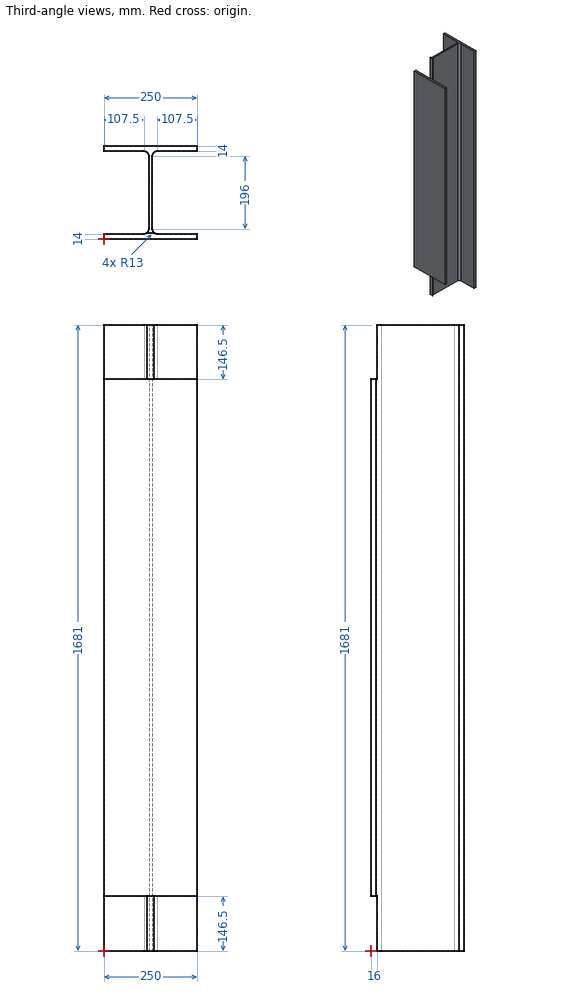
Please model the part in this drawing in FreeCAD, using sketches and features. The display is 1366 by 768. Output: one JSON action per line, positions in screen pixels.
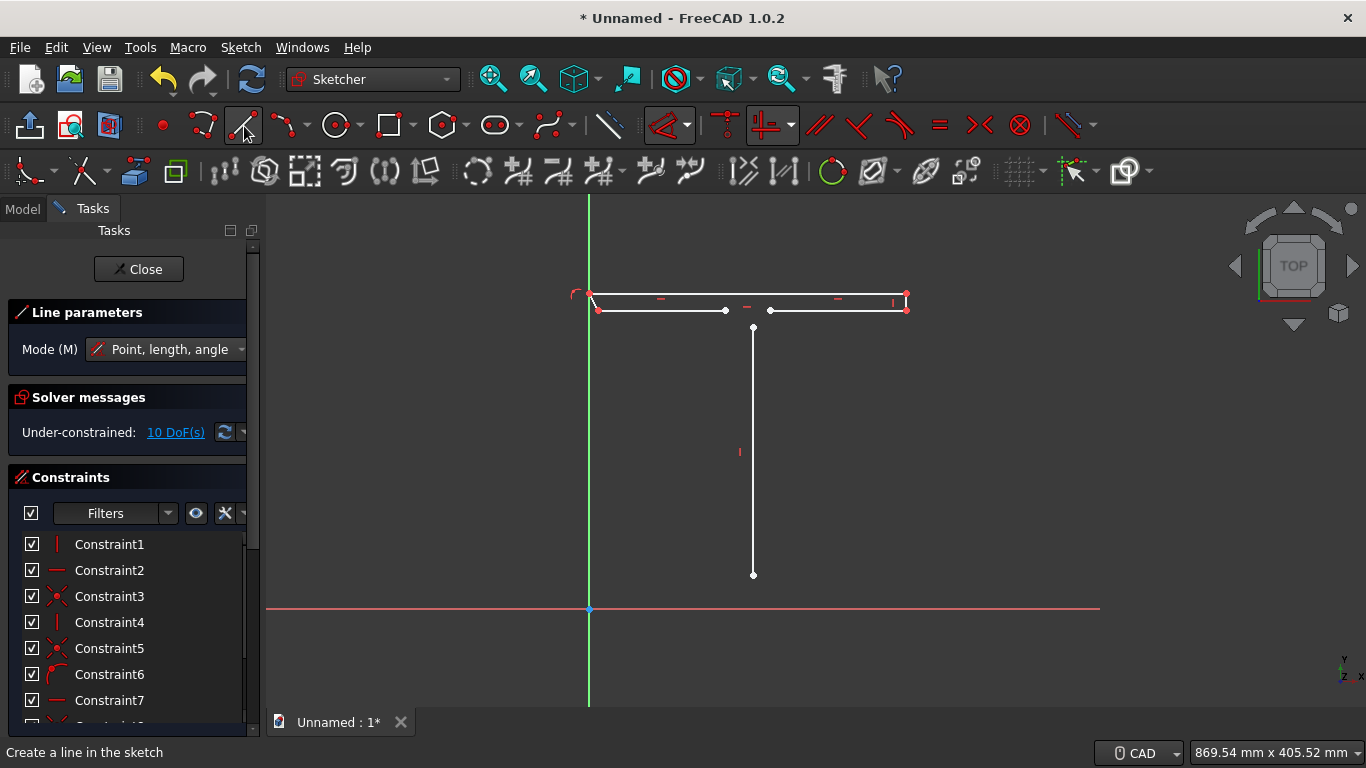
{"action": "scroll", "coordinate": [742, 327], "scroll_direction": "up", "scroll_amount": 2}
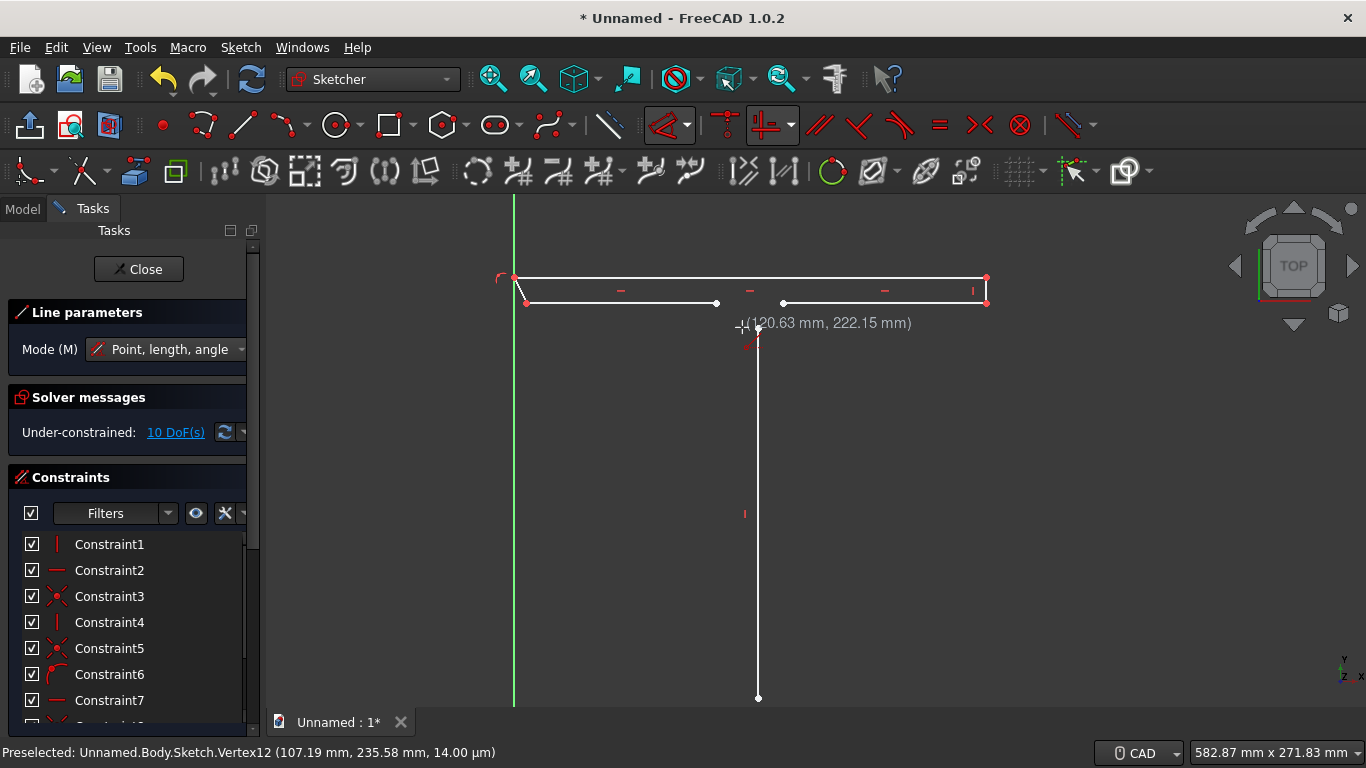
{"action": "left_click", "coordinate": [742, 327]}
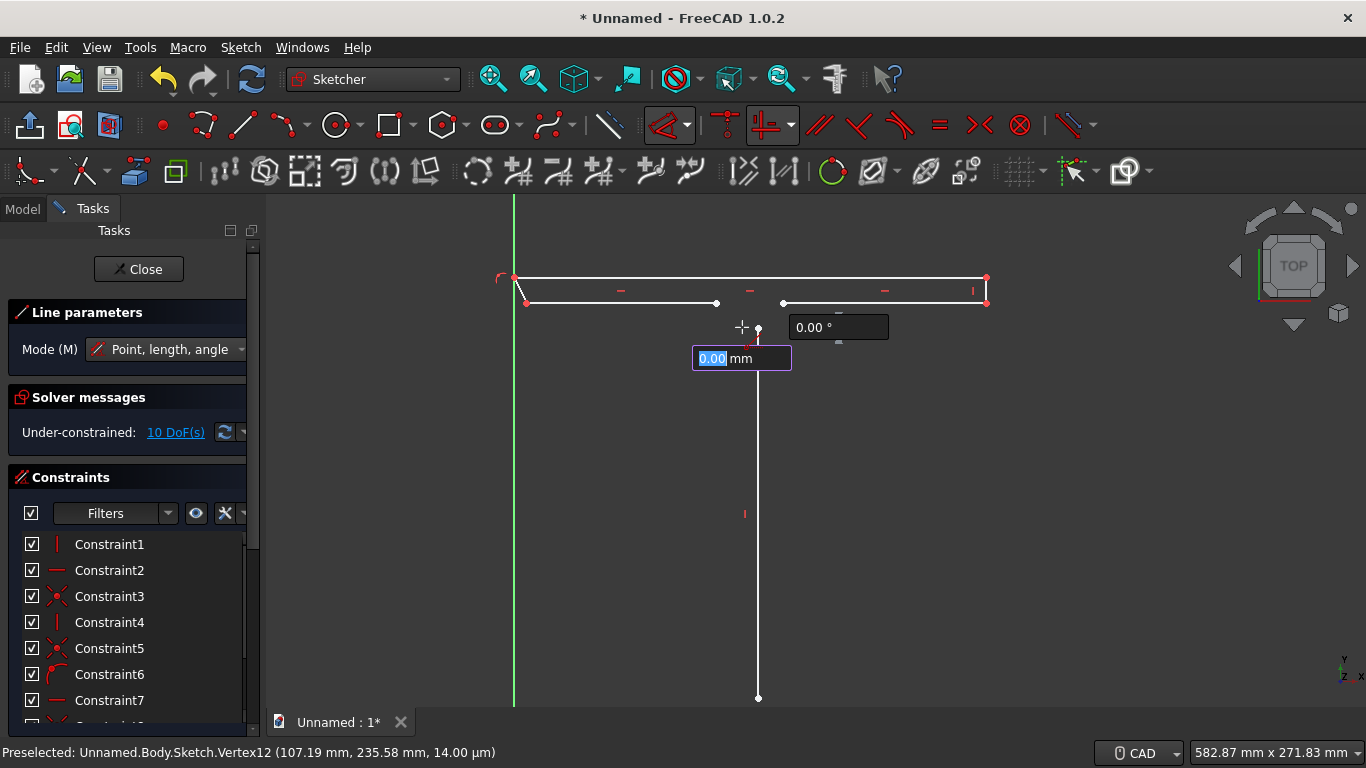
{"action": "scroll", "coordinate": [742, 326], "scroll_direction": "down", "scroll_amount": 2}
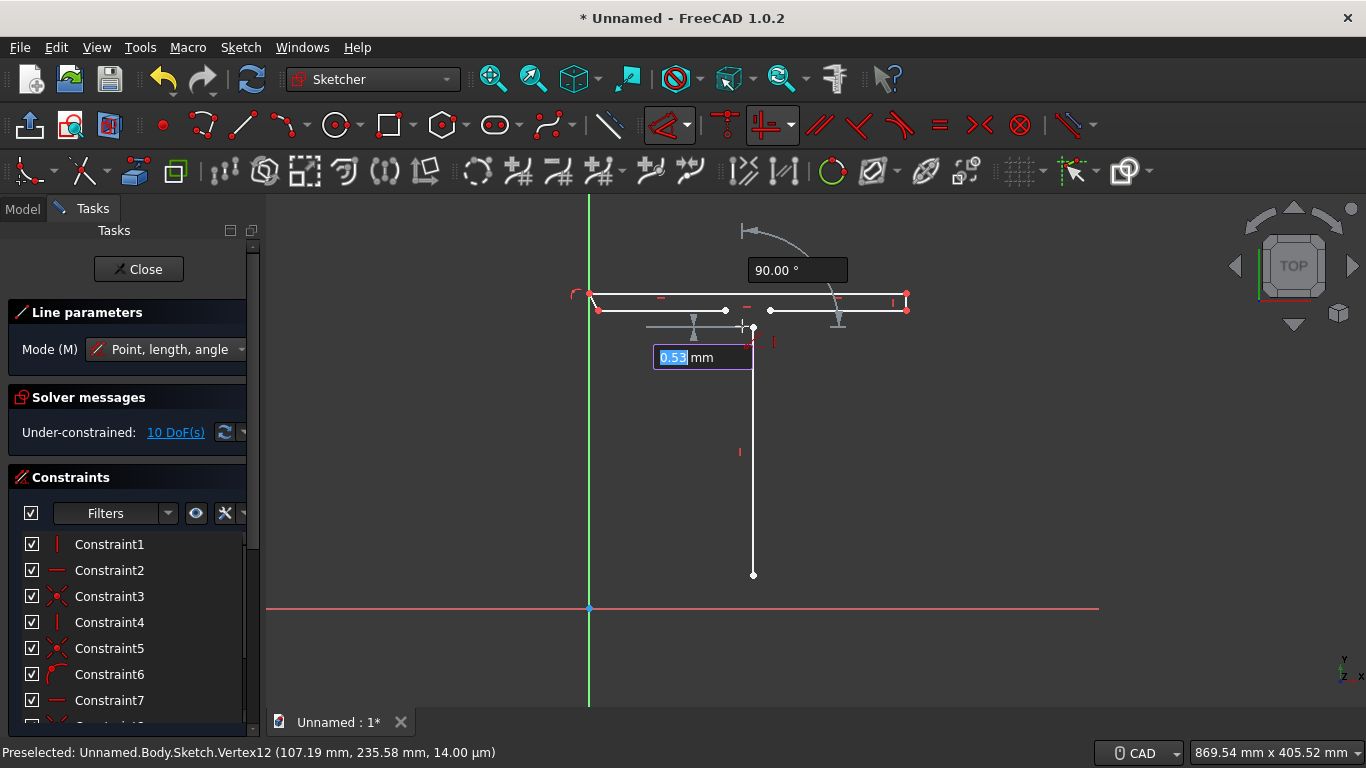
{"action": "scroll", "coordinate": [742, 575], "scroll_direction": "up", "scroll_amount": 2}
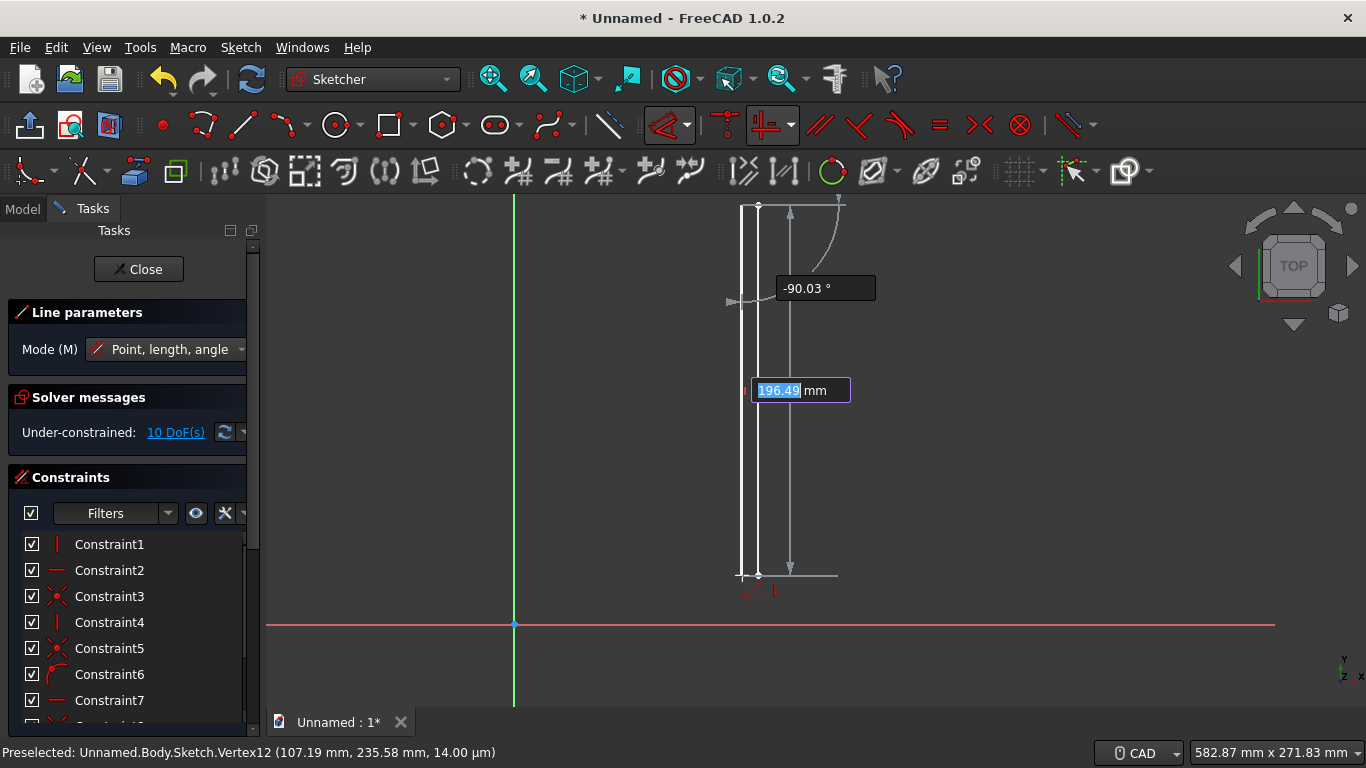
{"action": "left_click", "coordinate": [742, 574]}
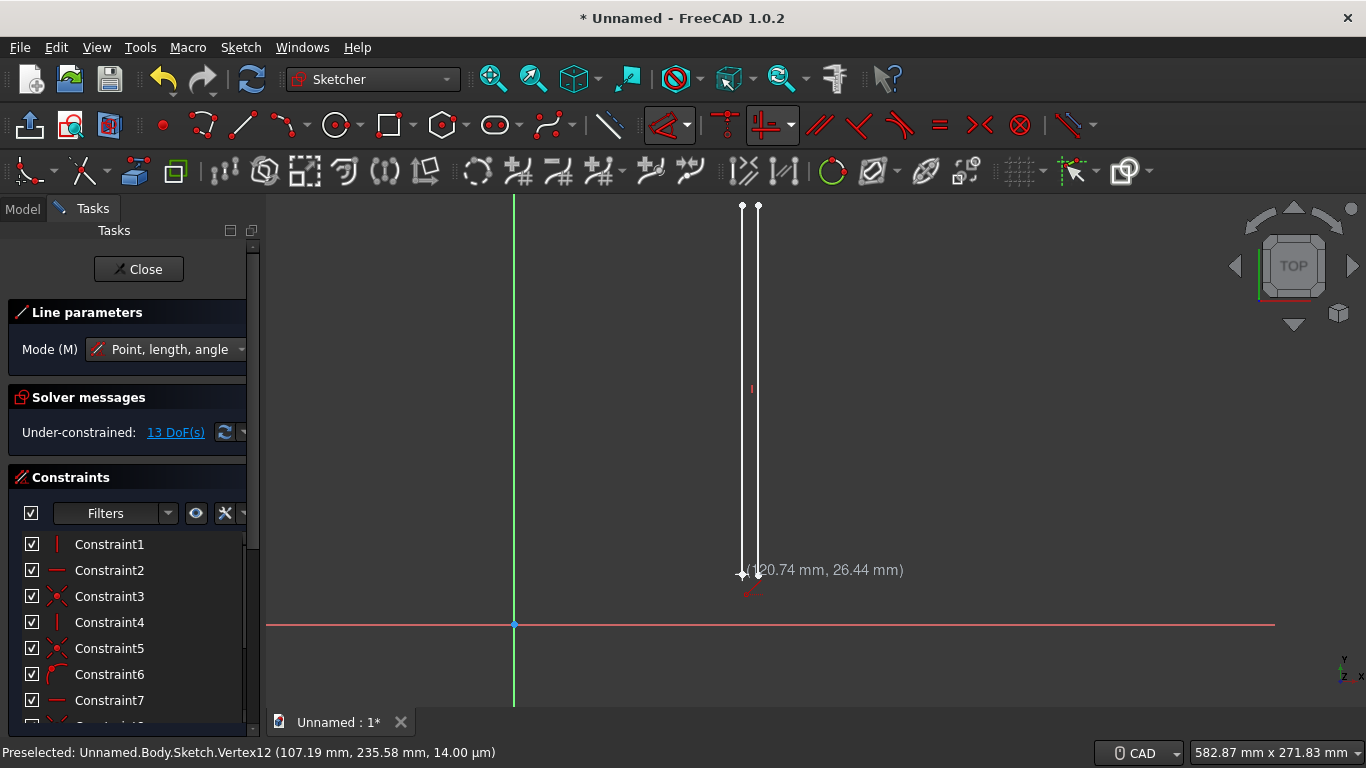
{"action": "left_click", "coordinate": [204, 126]}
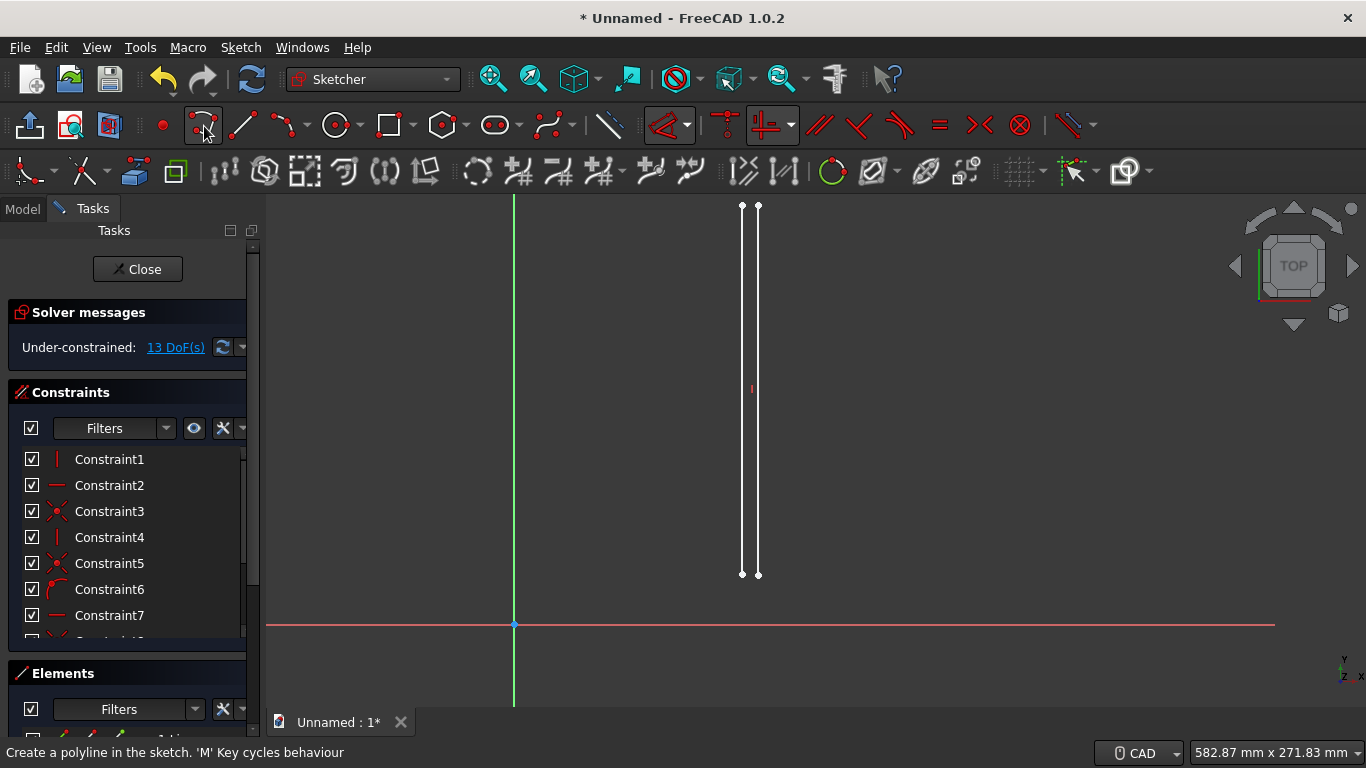
{"action": "left_click", "coordinate": [717, 598]}
{"action": "left_click", "coordinate": [514, 598]}
{"action": "left_click", "coordinate": [514, 625]}
{"action": "left_click", "coordinate": [986, 616]}
{"action": "left_click", "coordinate": [986, 598]}
{"action": "left_click", "coordinate": [783, 598]}
{"action": "right_click", "coordinate": [783, 598]}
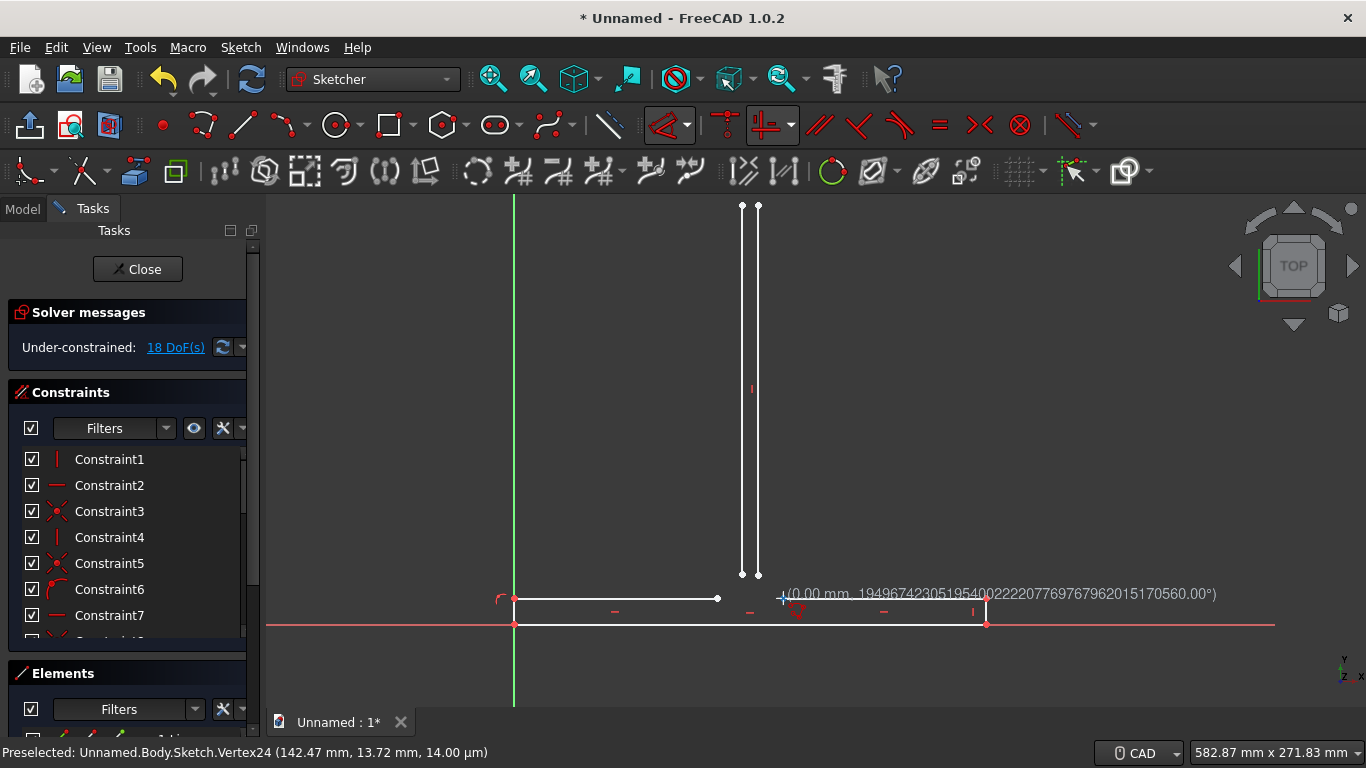
{"action": "left_click", "coordinate": [284, 126]}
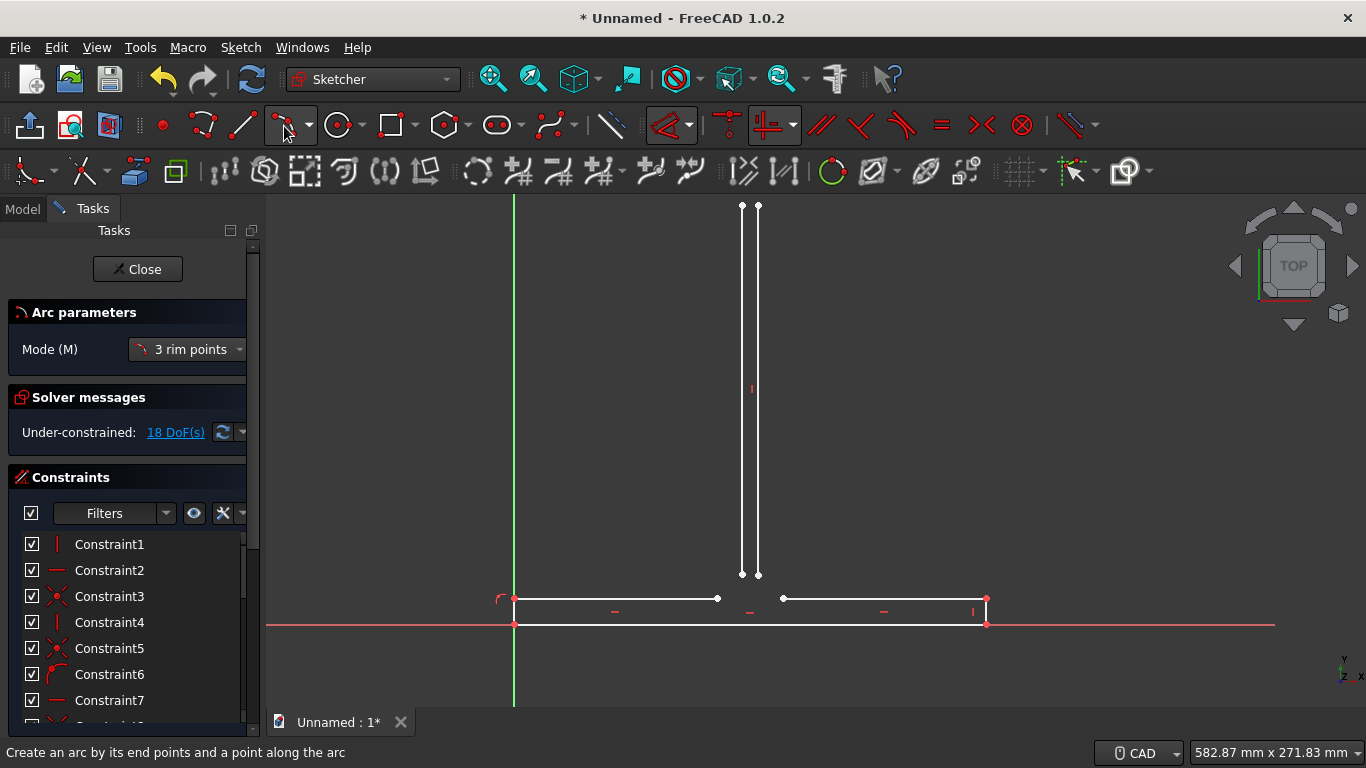
{"action": "scroll", "coordinate": [742, 576], "scroll_direction": "down", "scroll_amount": 2}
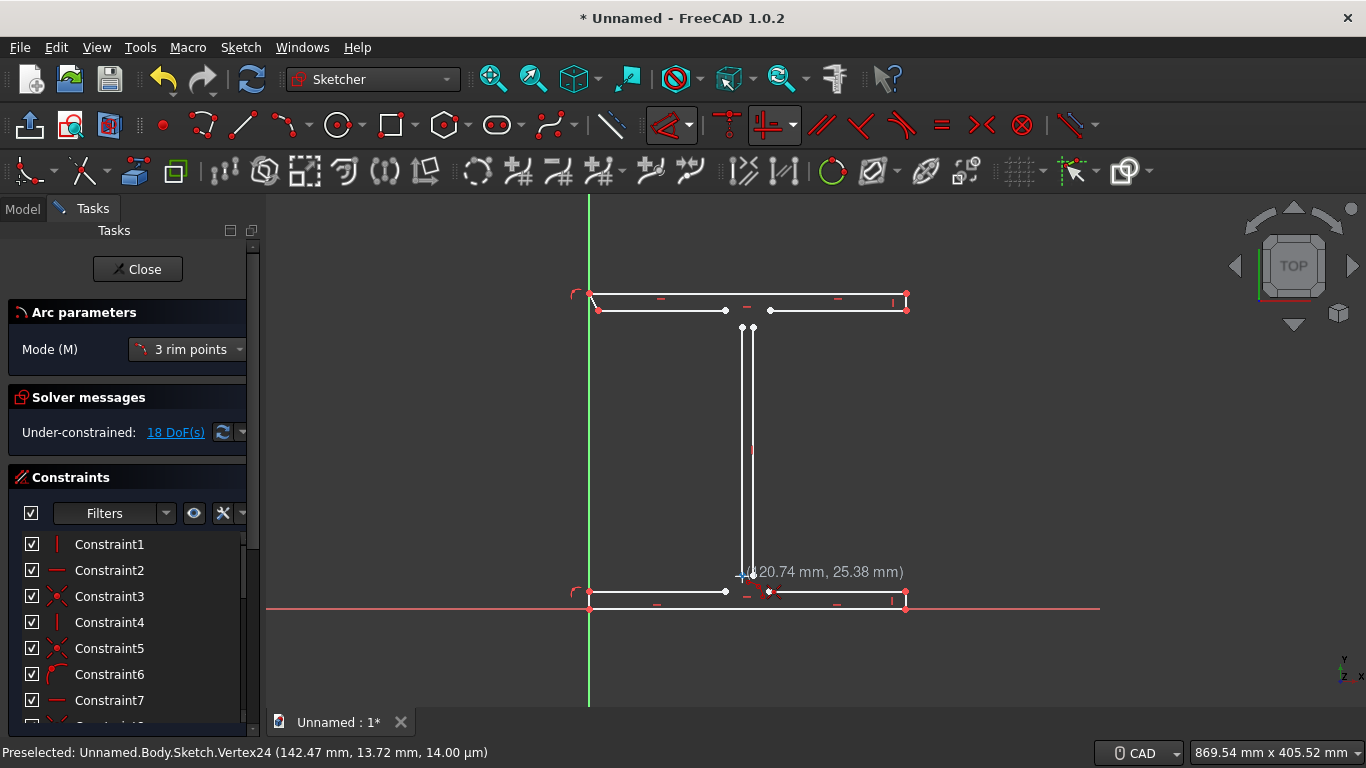
{"action": "scroll", "coordinate": [753, 327], "scroll_direction": "up", "scroll_amount": 2}